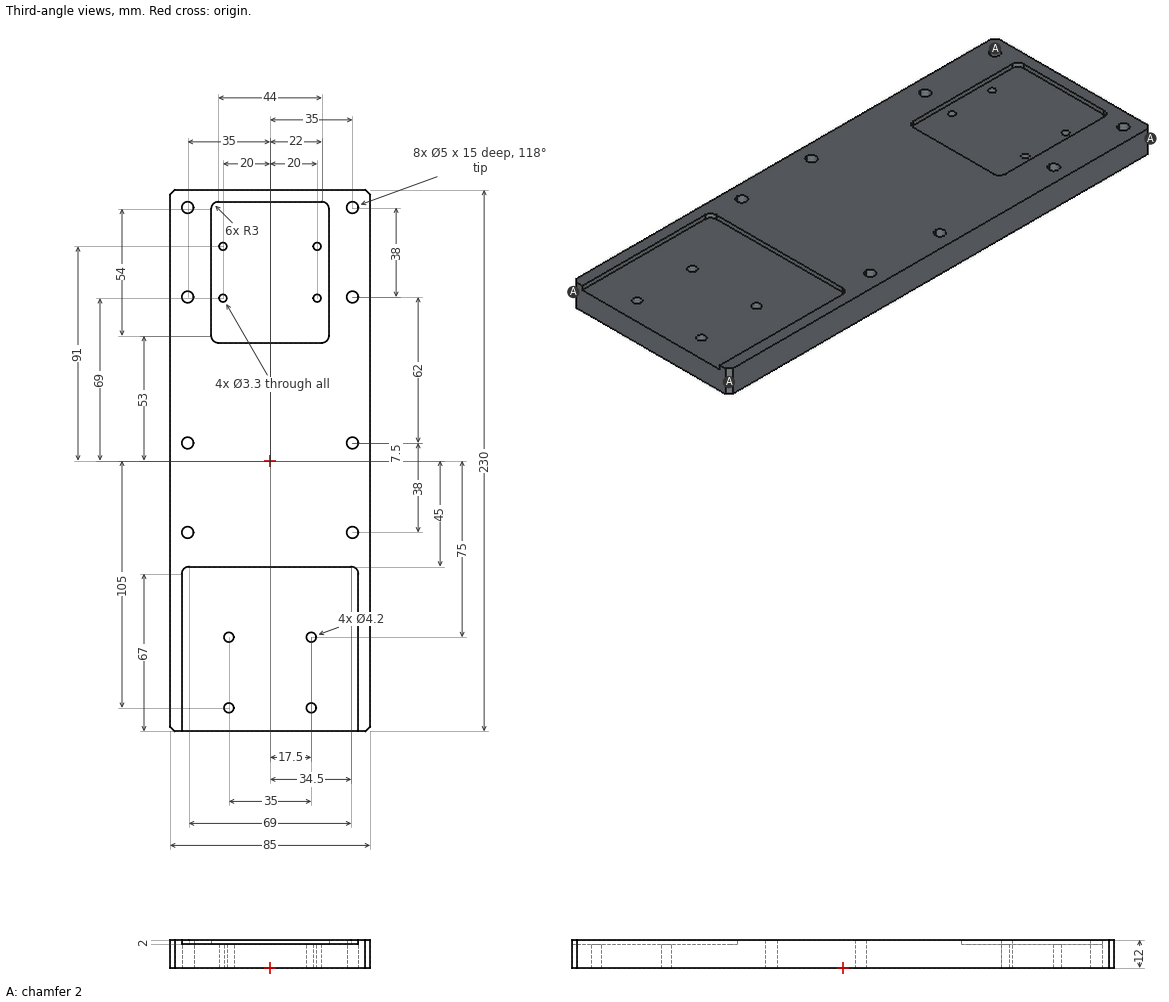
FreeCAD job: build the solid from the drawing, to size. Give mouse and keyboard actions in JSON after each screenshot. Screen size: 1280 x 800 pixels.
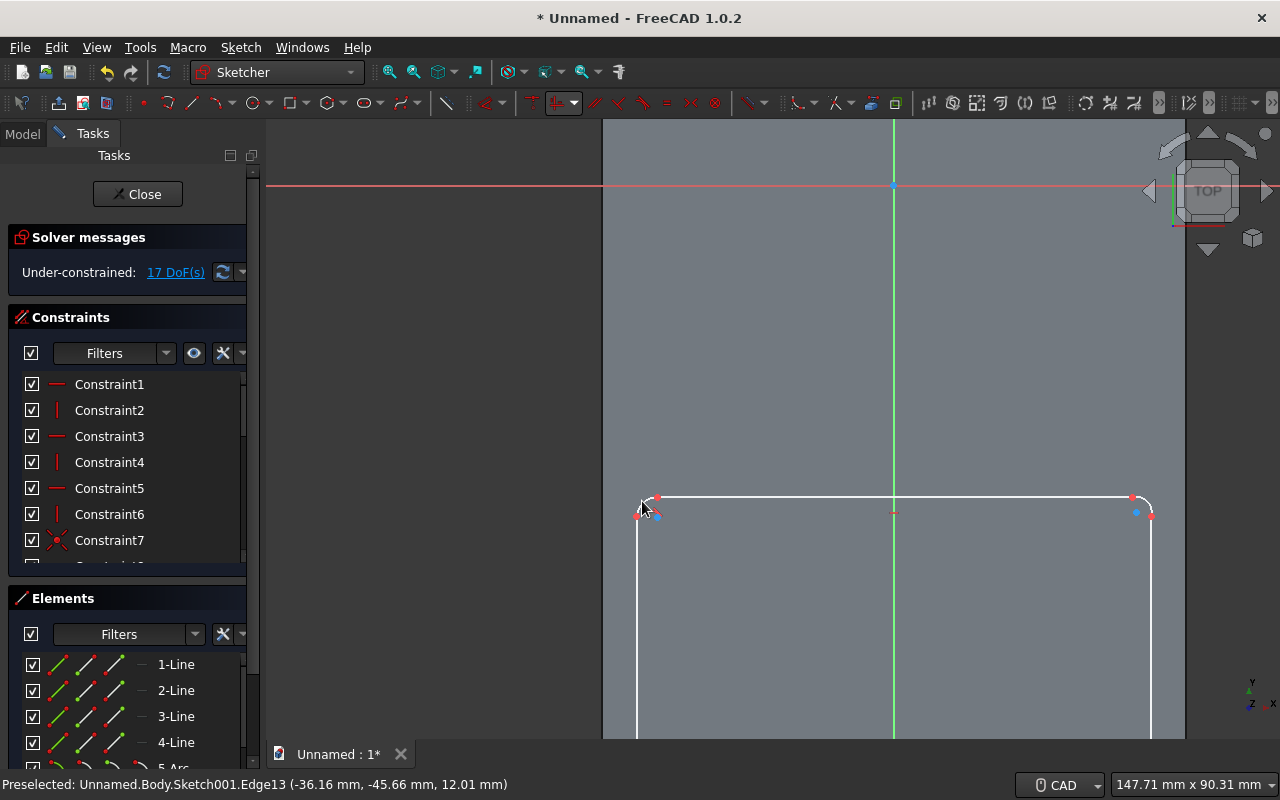
{"action": "scroll", "coordinate": [643, 503], "scroll_direction": "down", "scroll_amount": 7}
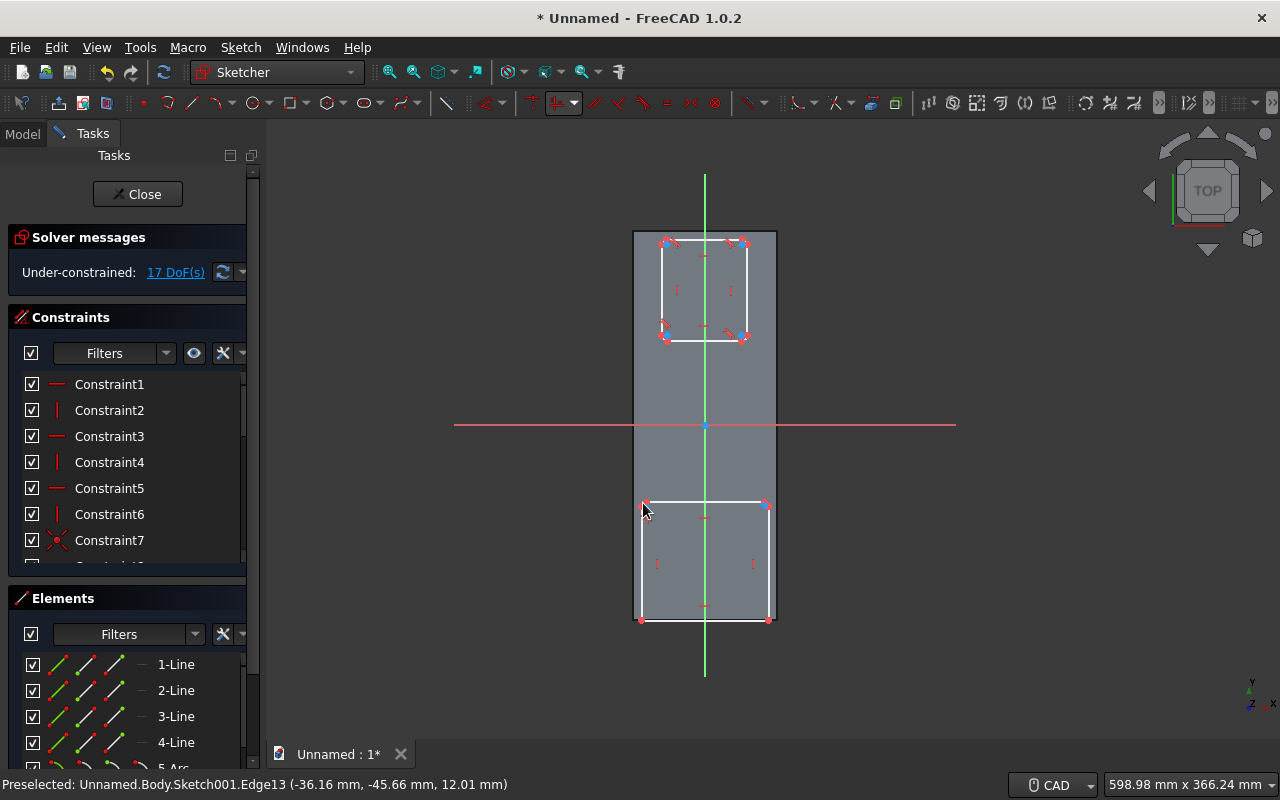
{"action": "left_click", "coordinate": [729, 502]}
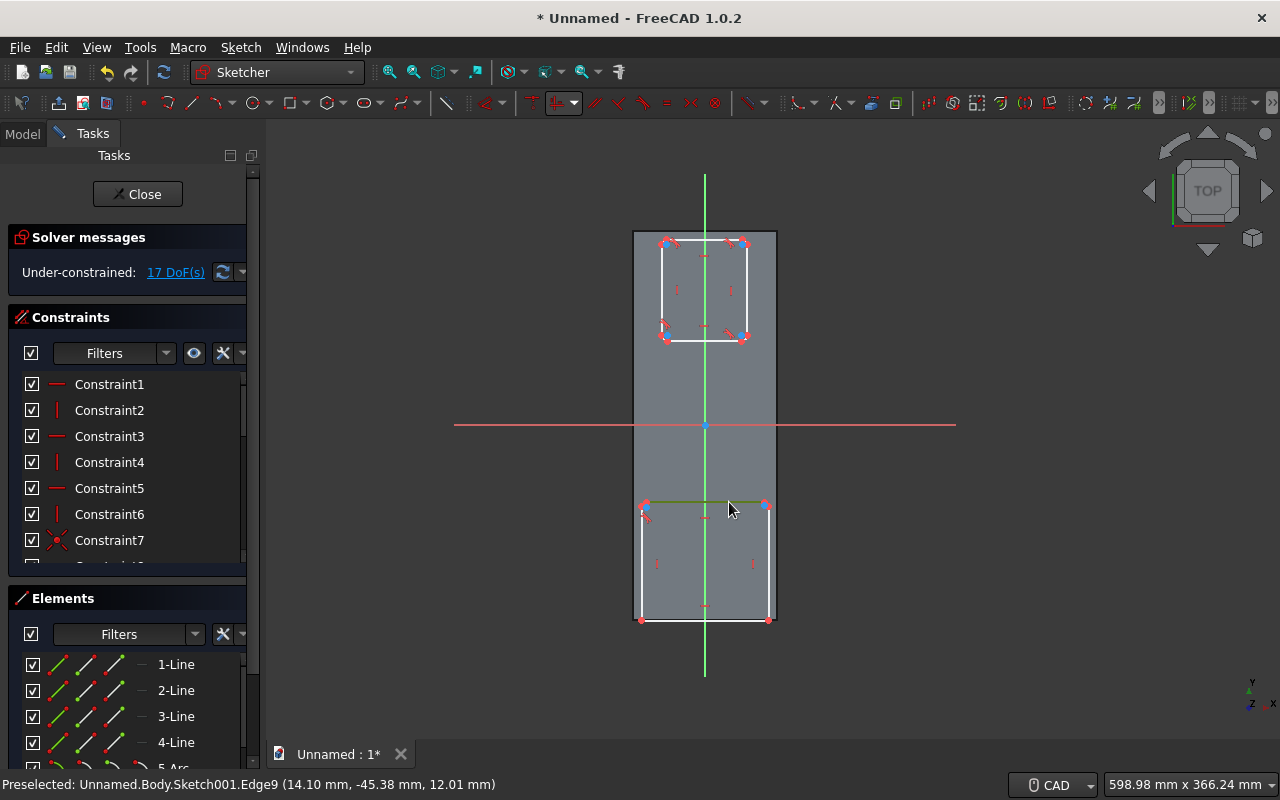
{"action": "scroll", "coordinate": [768, 503], "scroll_direction": "up", "scroll_amount": 7}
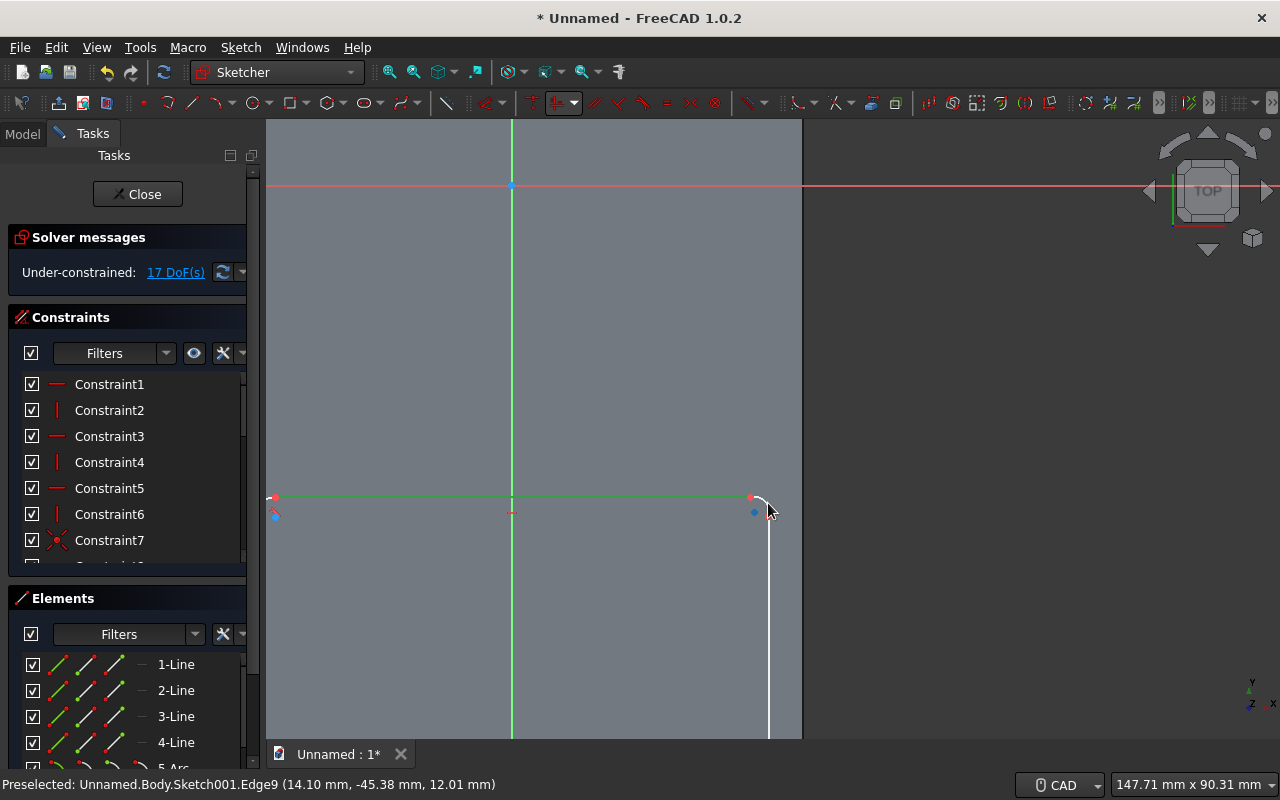
{"action": "left_click", "coordinate": [765, 501]}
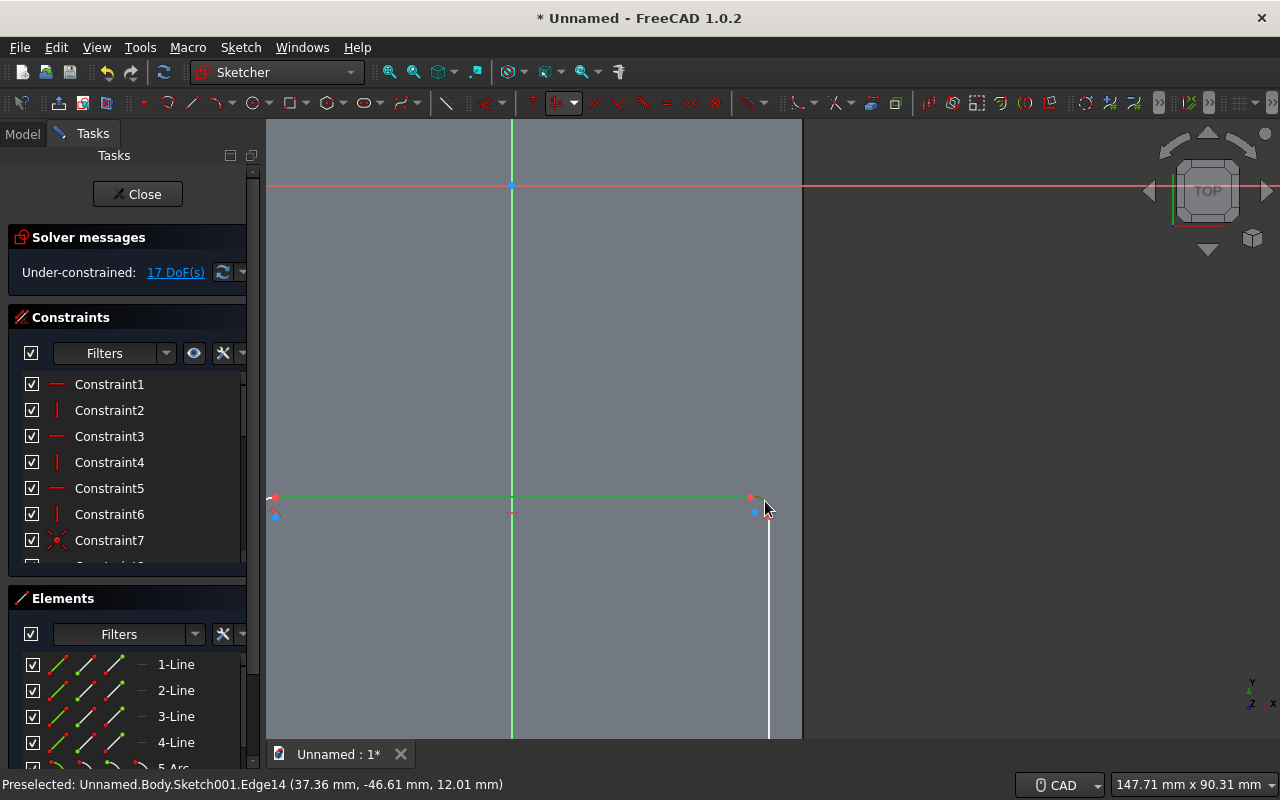
{"action": "key", "text": "t"}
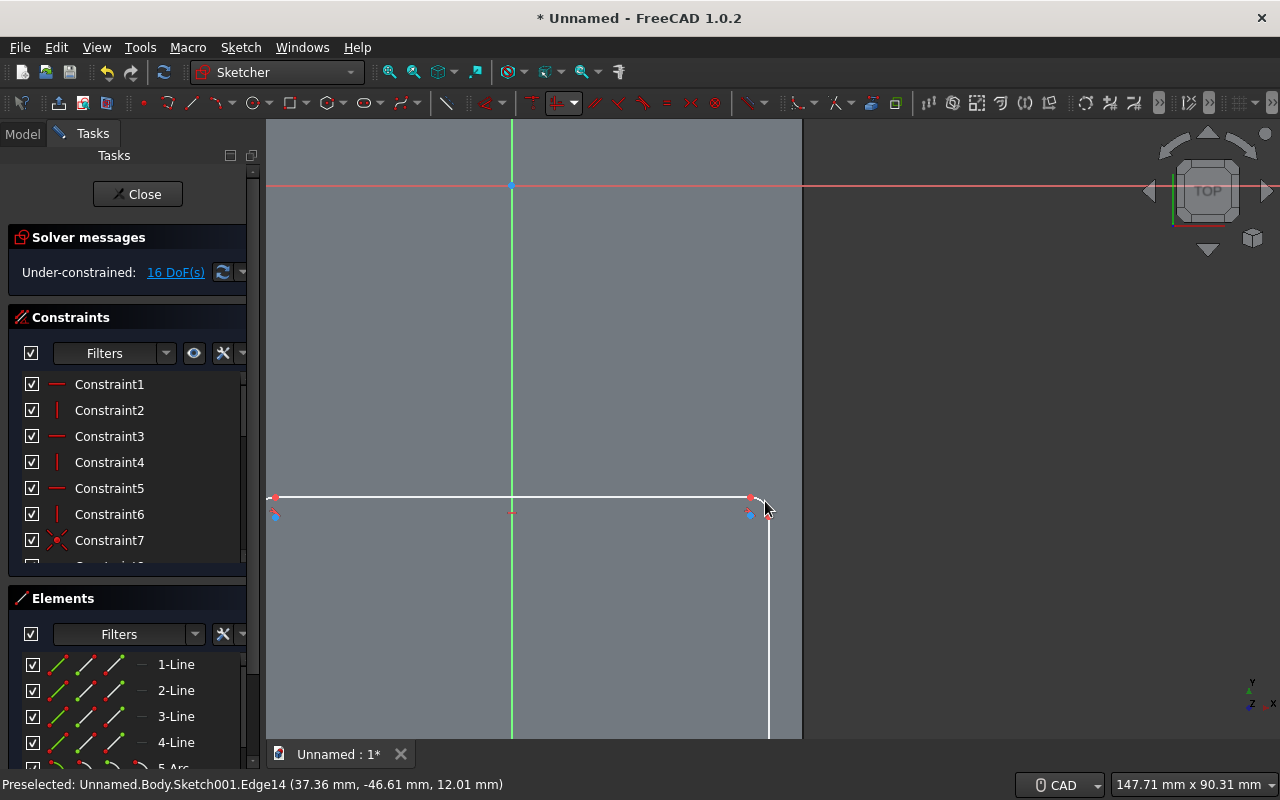
{"action": "scroll", "coordinate": [768, 503], "scroll_direction": "down", "scroll_amount": 7}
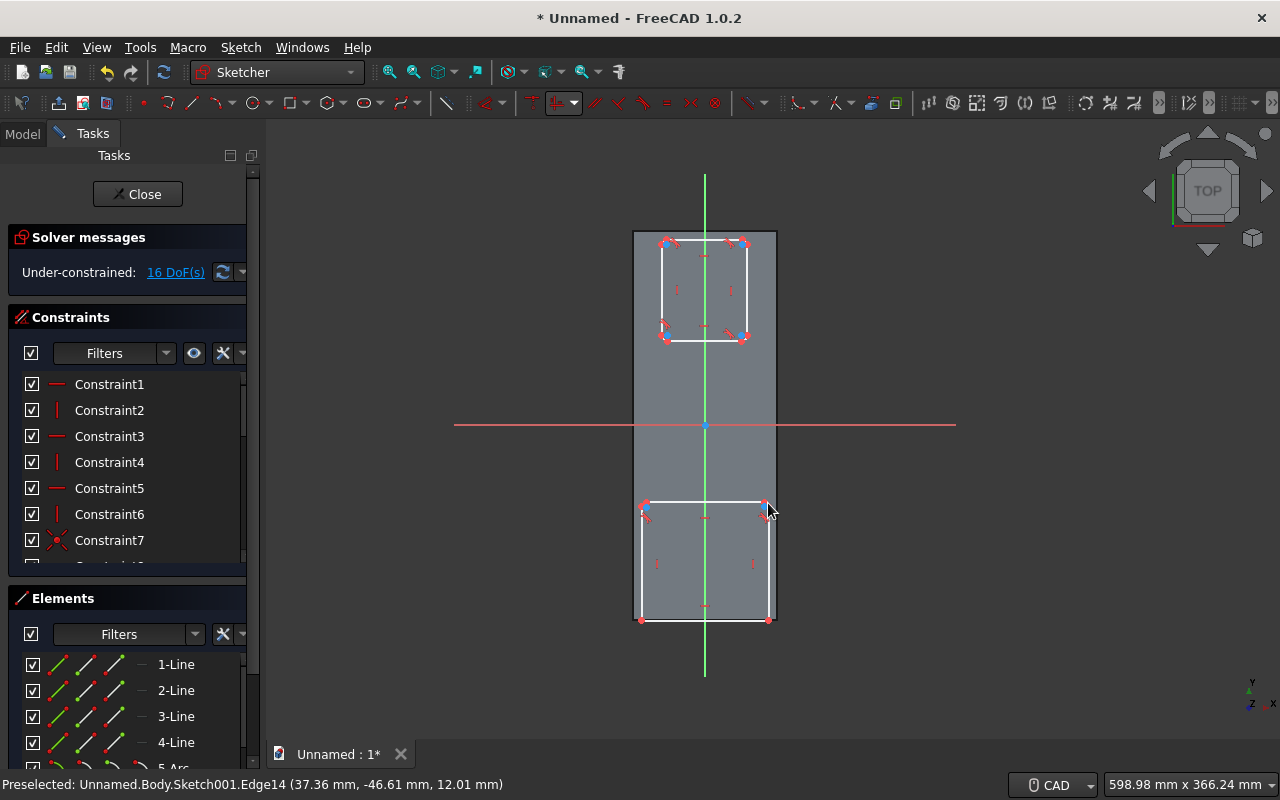
{"action": "left_click", "coordinate": [642, 541]}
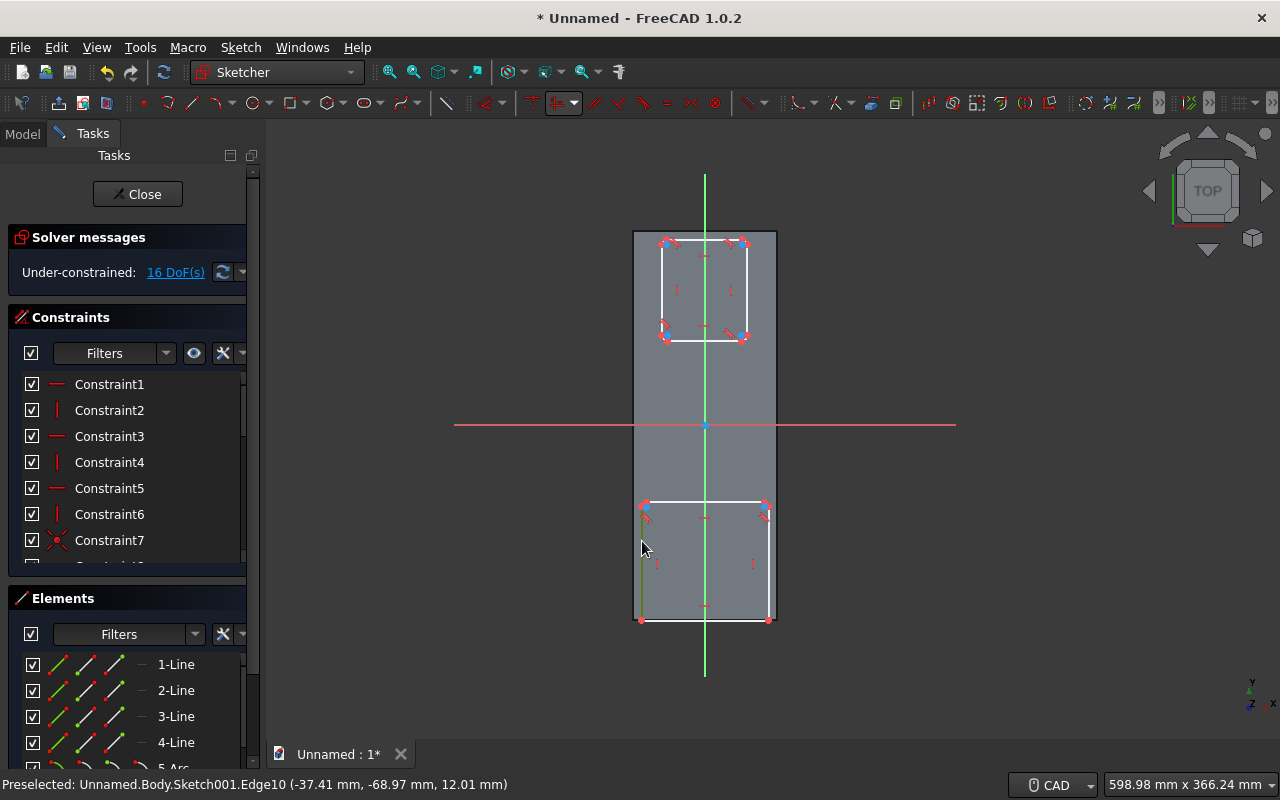
{"action": "scroll", "coordinate": [643, 503], "scroll_direction": "up", "scroll_amount": 7}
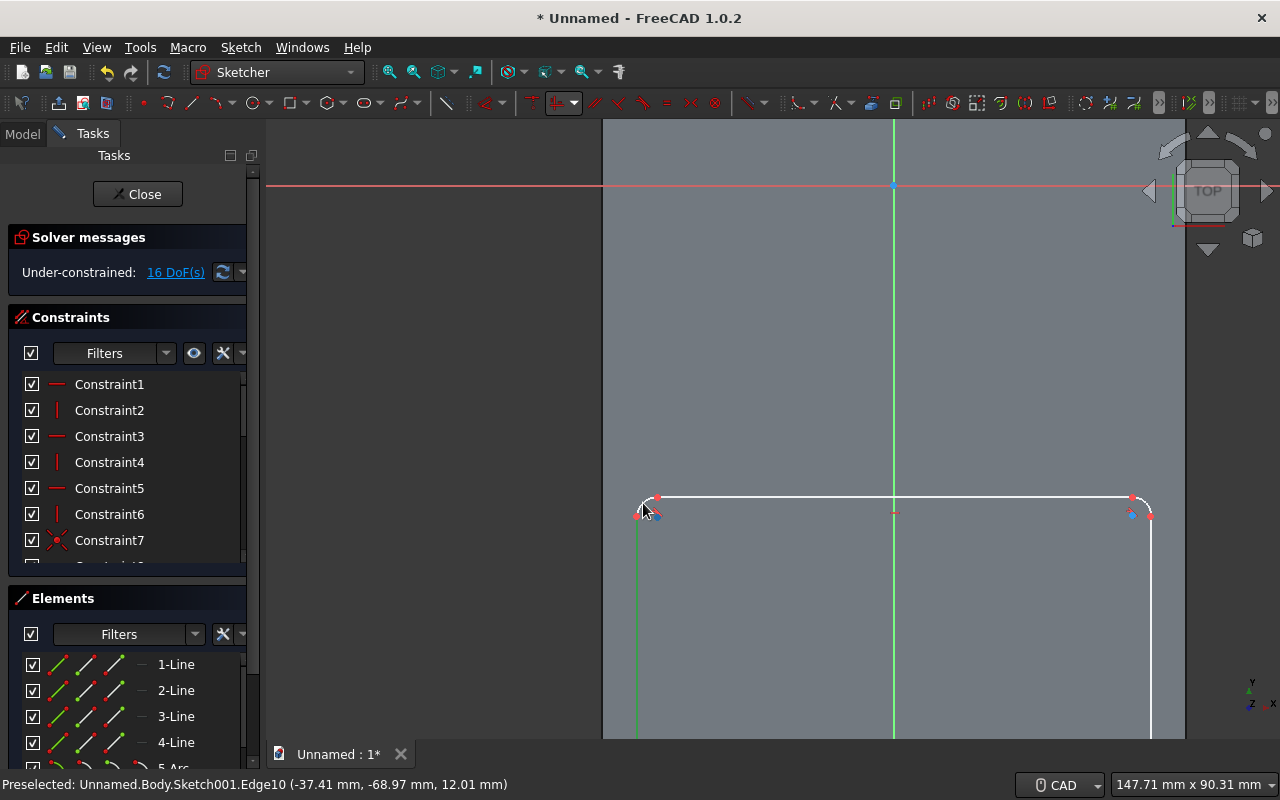
{"action": "left_click", "coordinate": [643, 503]}